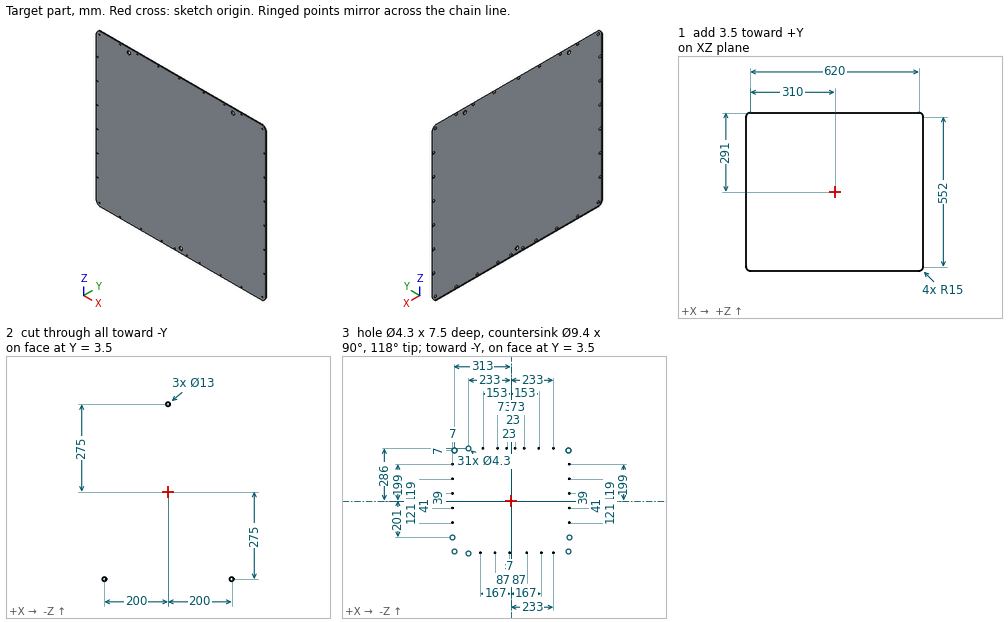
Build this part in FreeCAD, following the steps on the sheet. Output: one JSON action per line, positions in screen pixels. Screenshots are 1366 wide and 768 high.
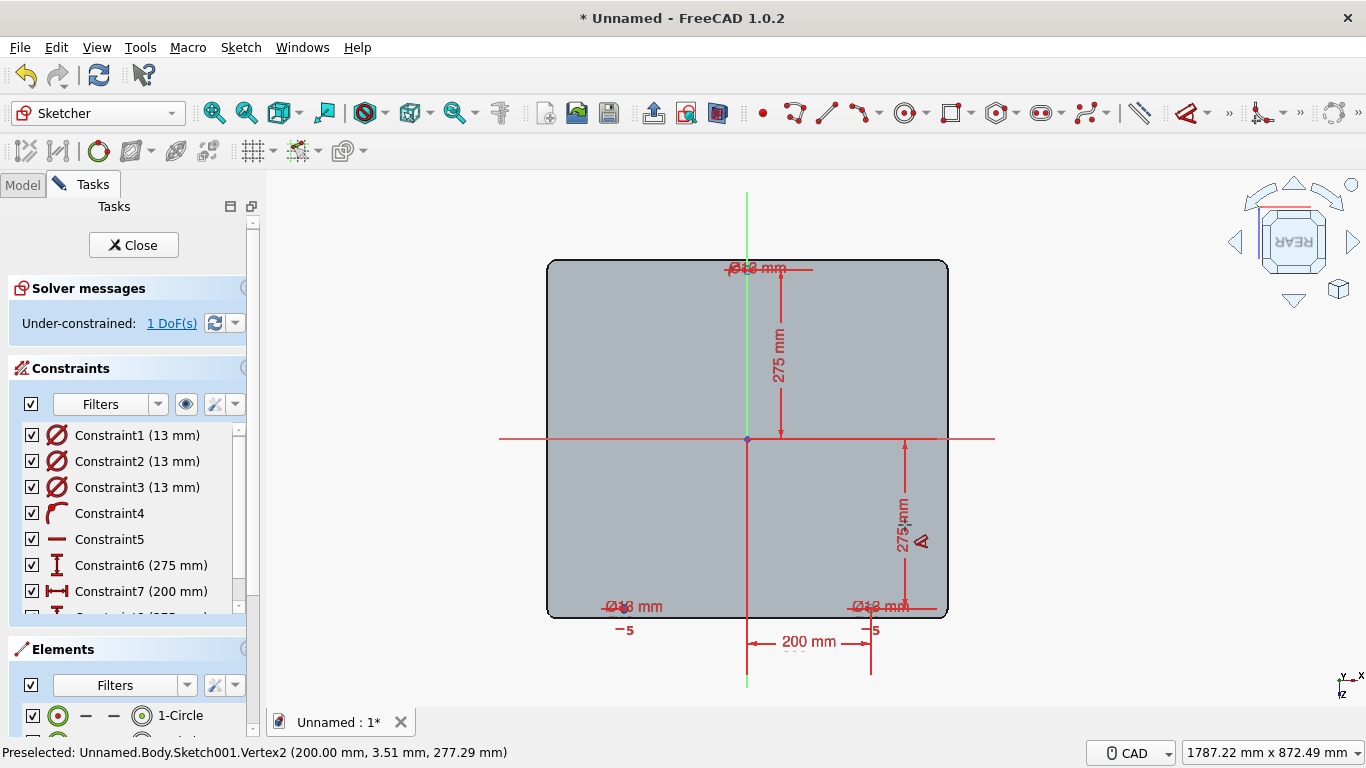
{"action": "left_click", "coordinate": [624, 609]}
{"action": "left_click", "coordinate": [686, 643]}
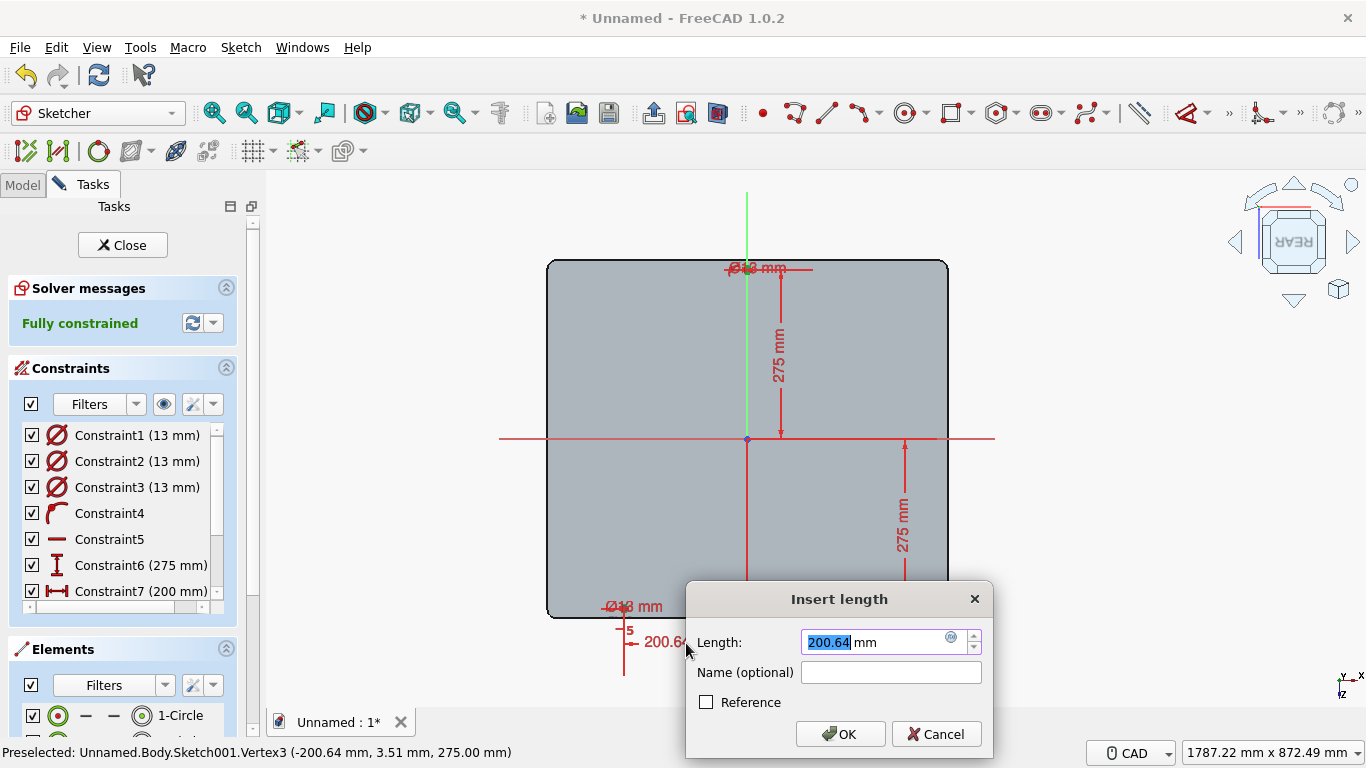
{"action": "type", "text": "200"}
{"action": "key", "text": "Return"}
{"action": "key", "text": "Escape"}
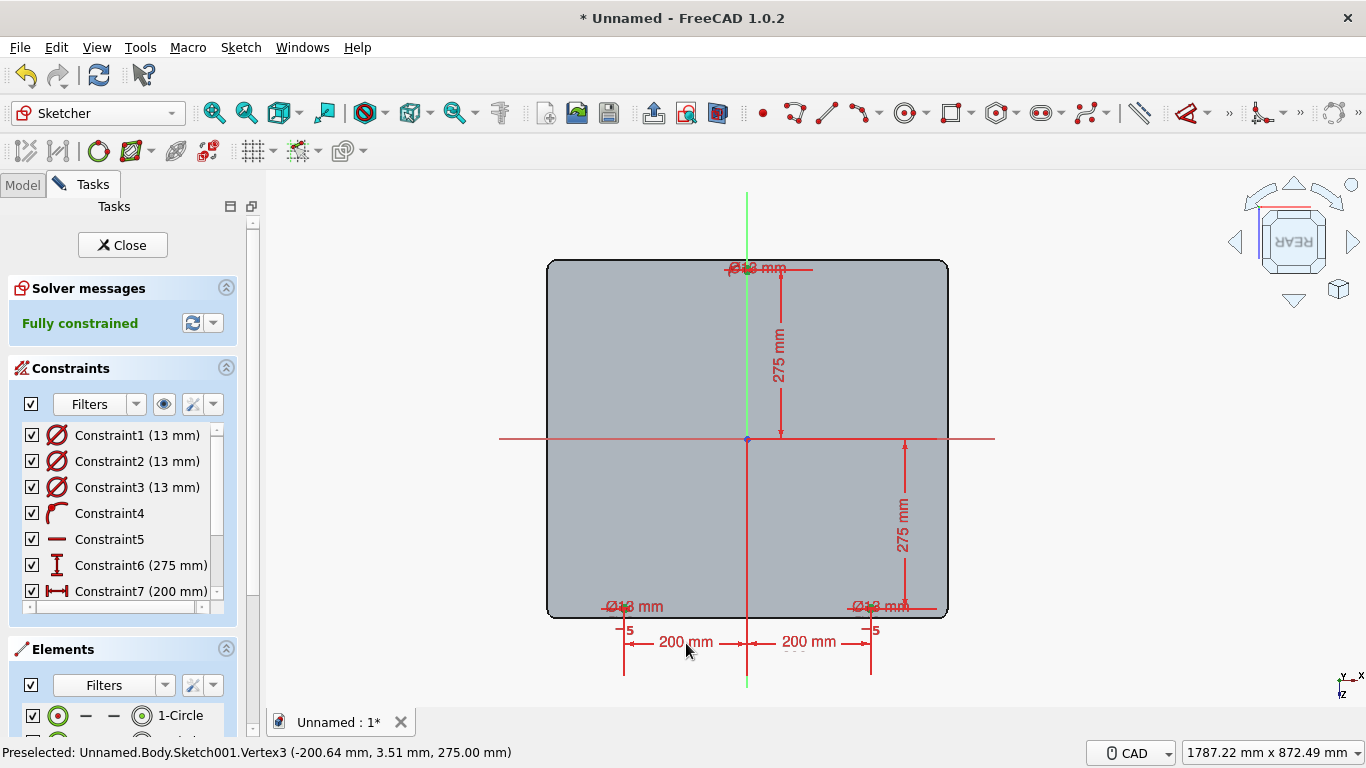
{"action": "left_click", "coordinate": [123, 245]}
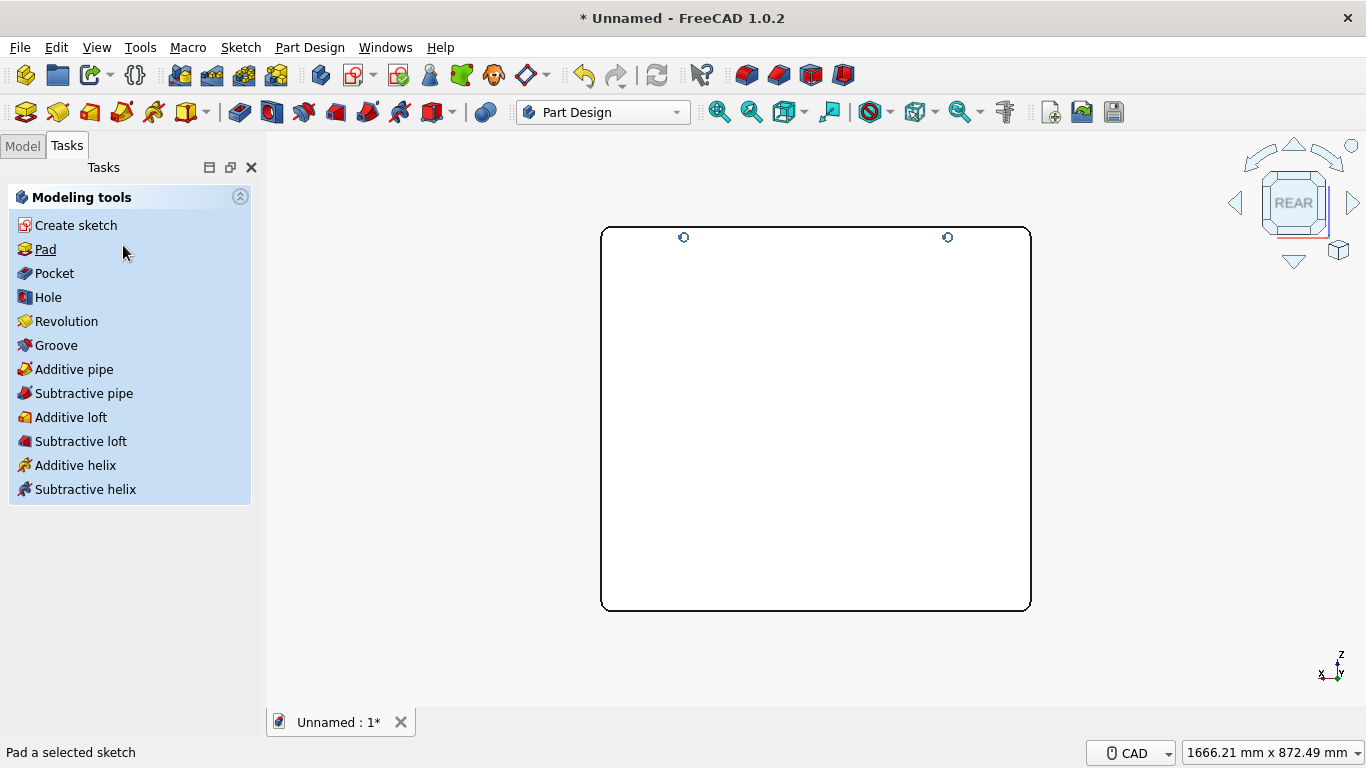
{"action": "left_click", "coordinate": [240, 112]}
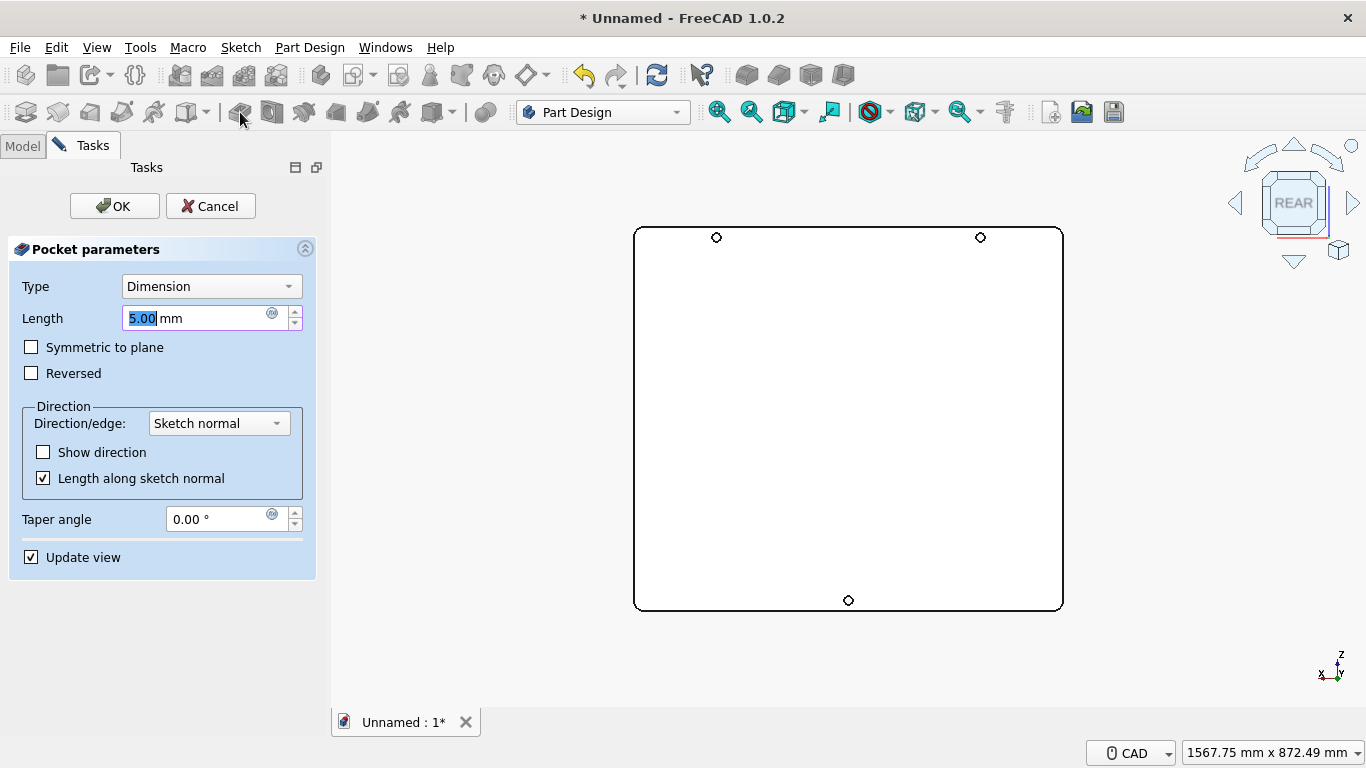
{"action": "left_click", "coordinate": [212, 286]}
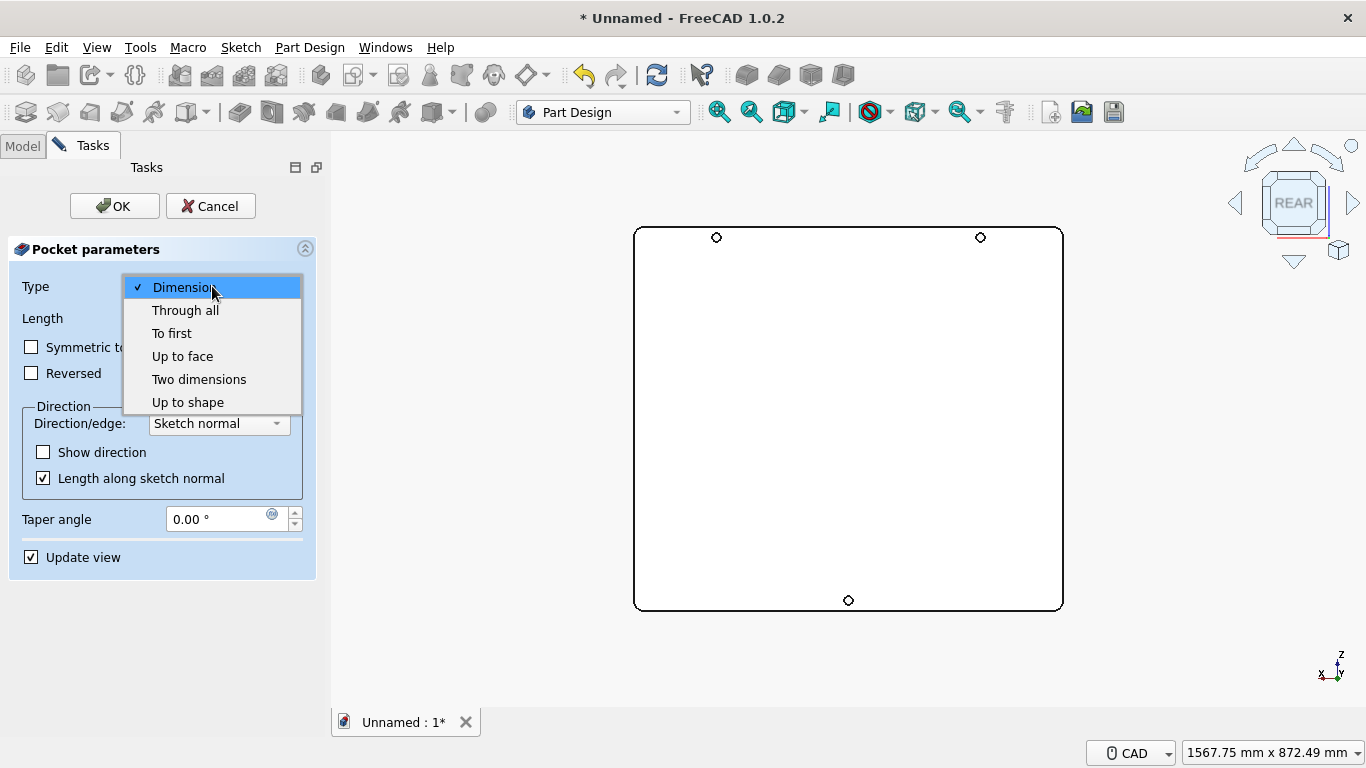
{"action": "left_click", "coordinate": [212, 310]}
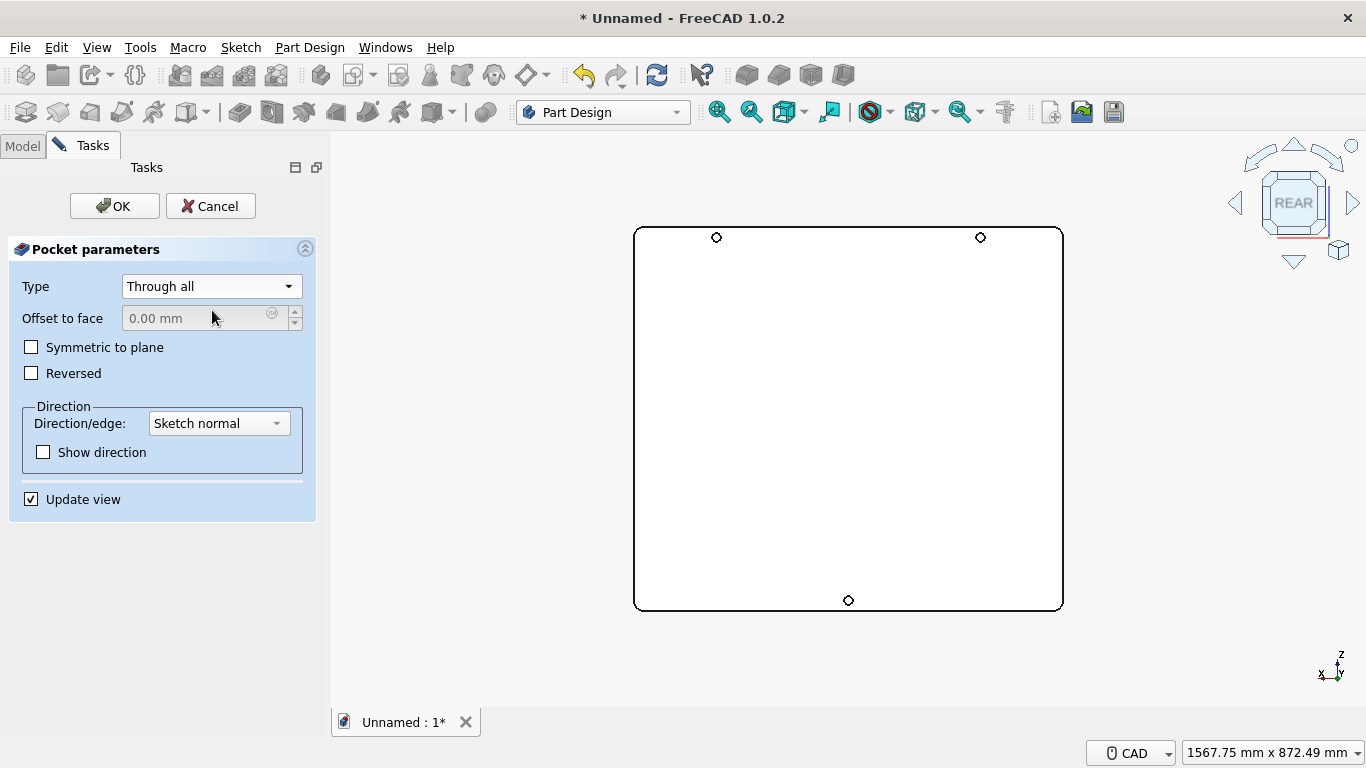
{"action": "left_click", "coordinate": [115, 206]}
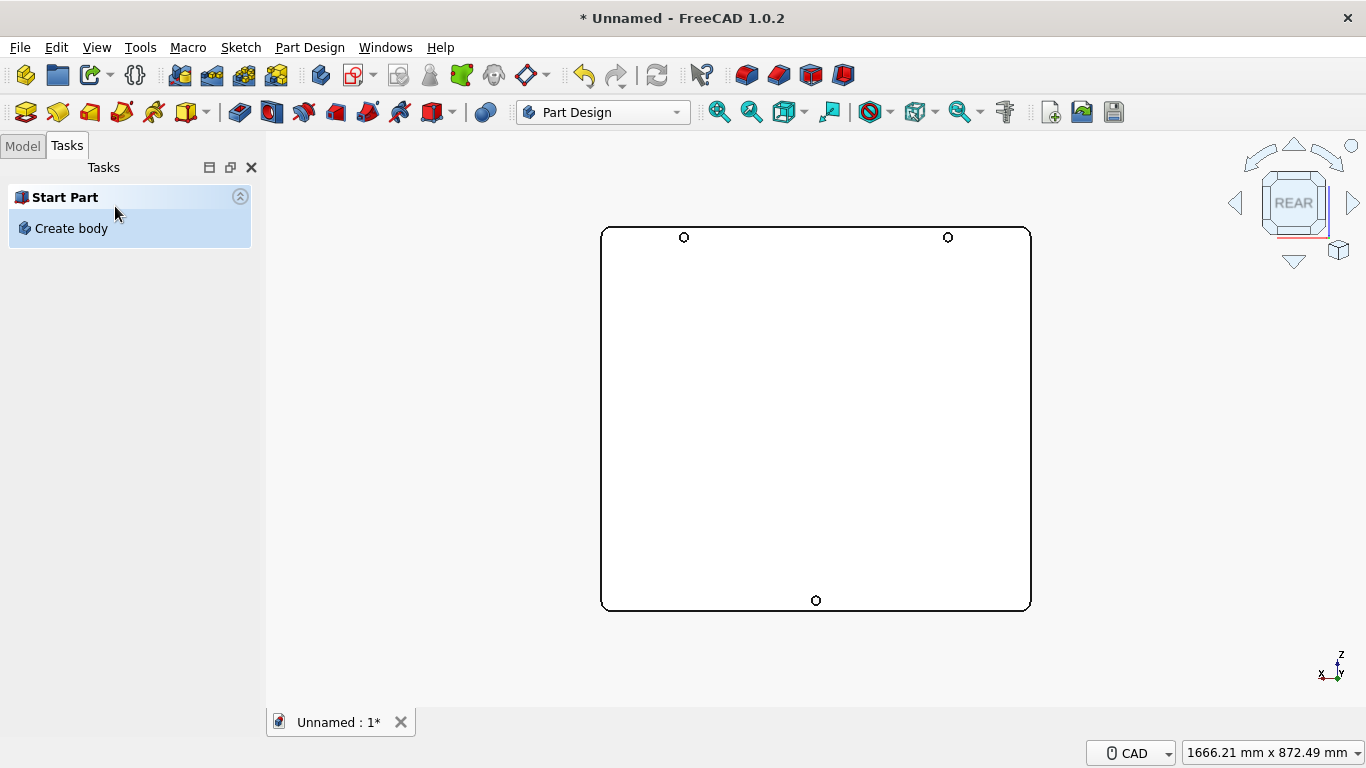
{"action": "left_click", "coordinate": [816, 418]}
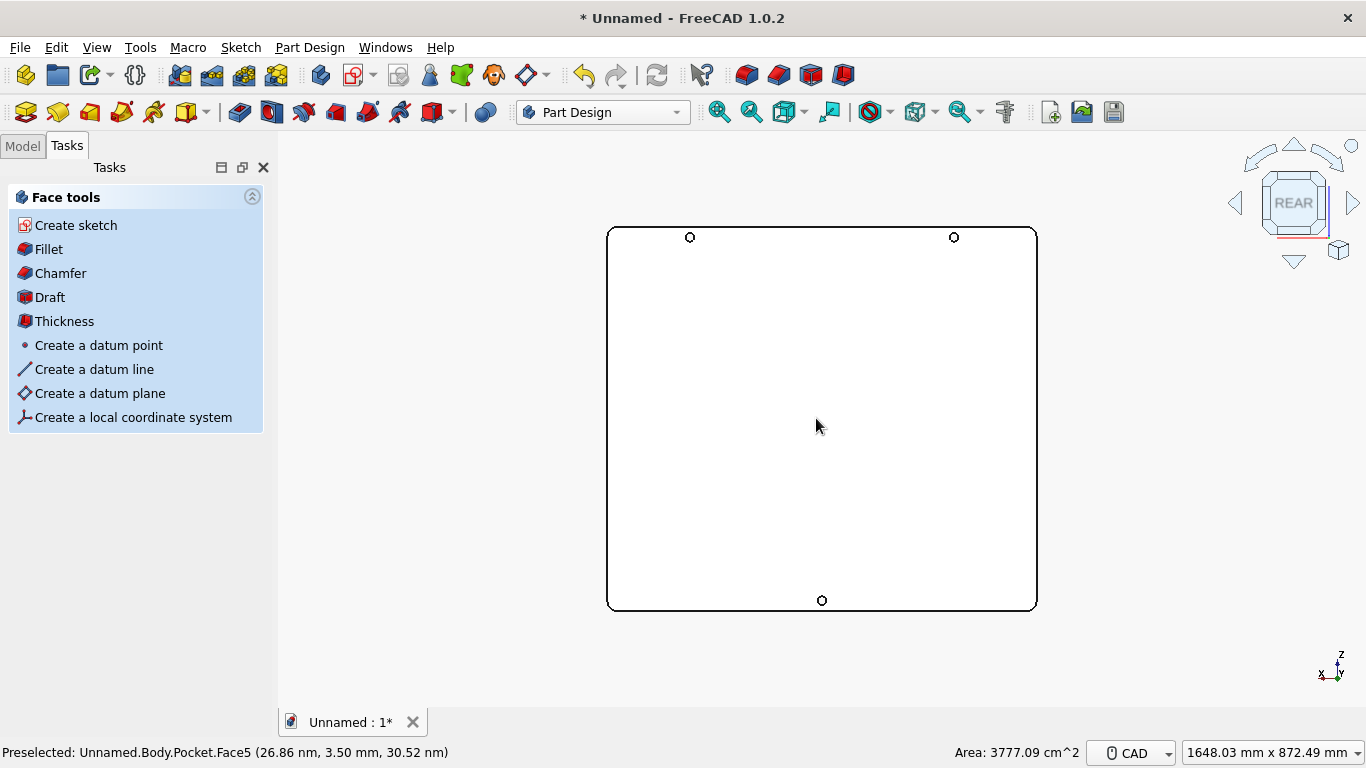
{"action": "left_click", "coordinate": [354, 76]}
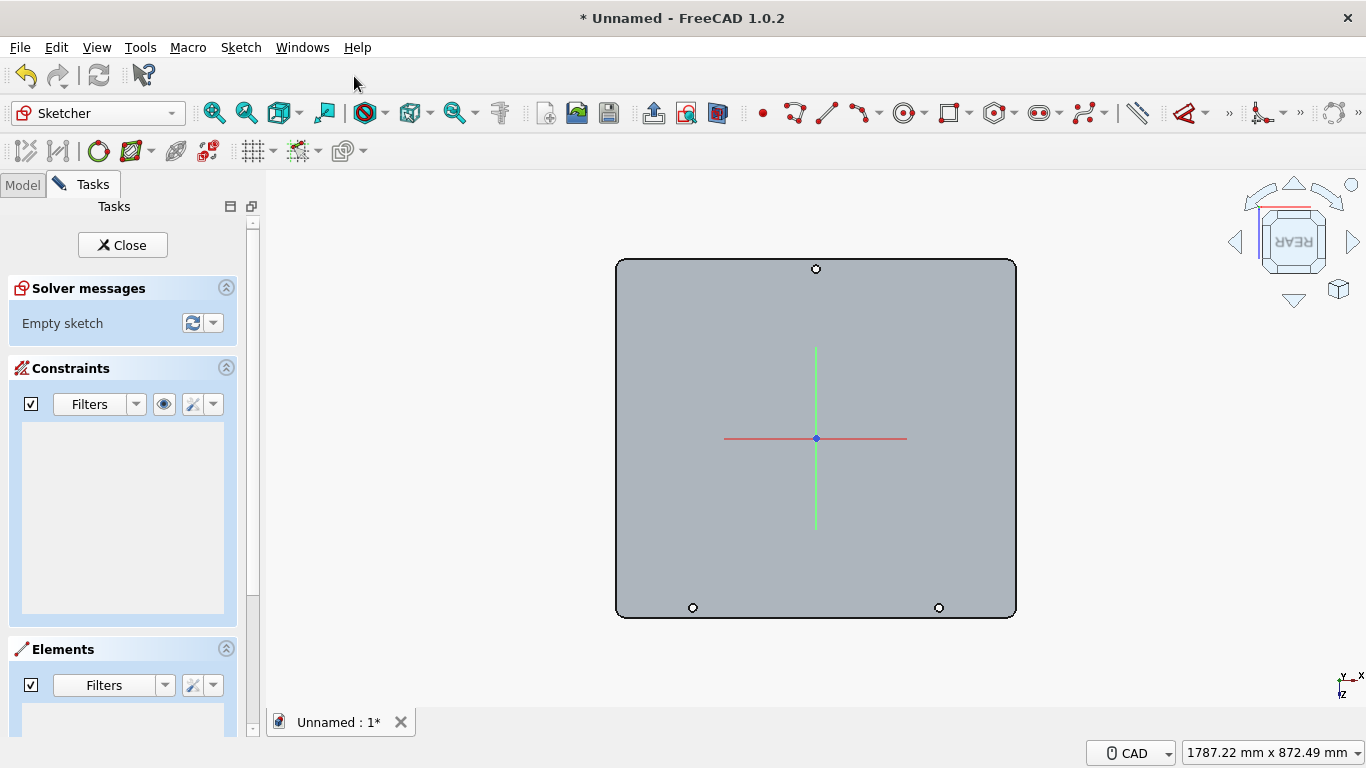
{"action": "left_click", "coordinate": [904, 114]}